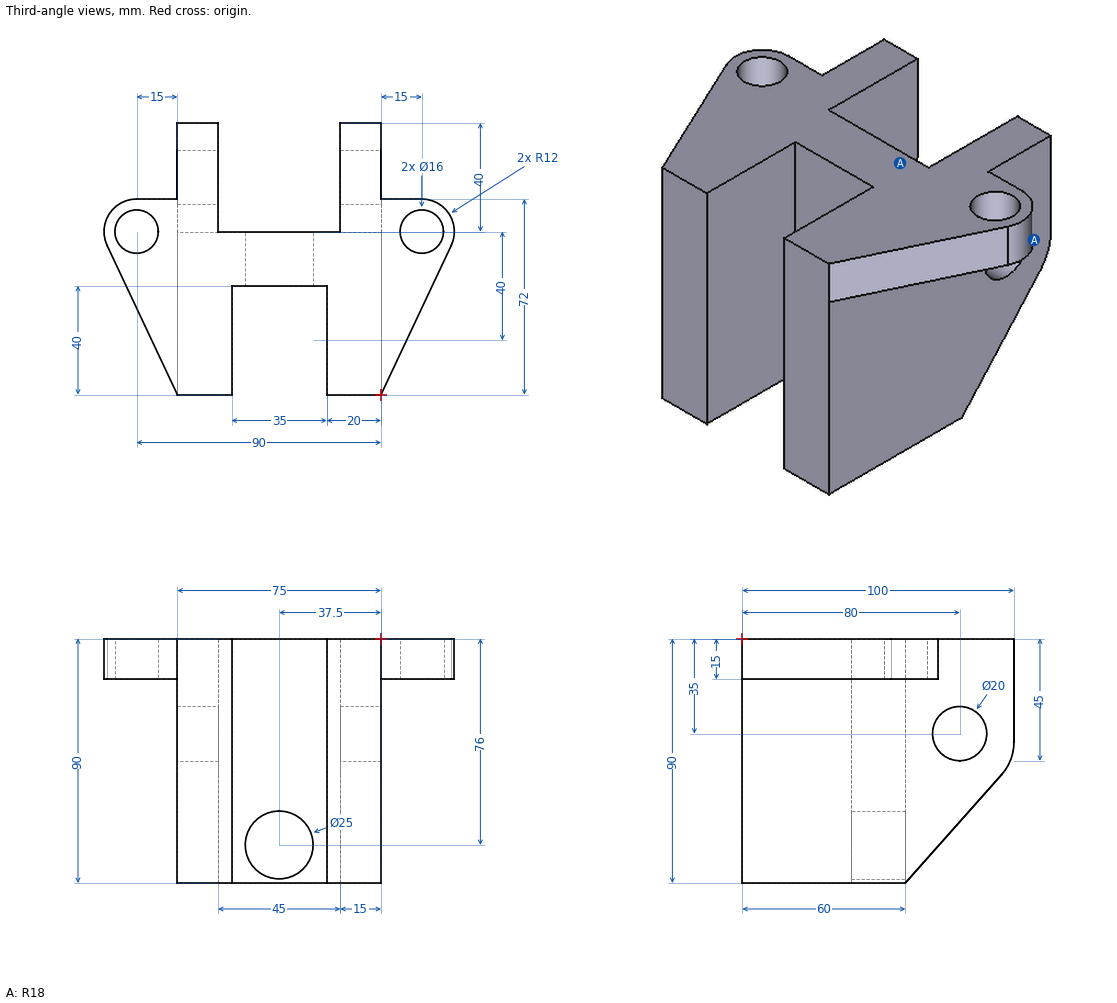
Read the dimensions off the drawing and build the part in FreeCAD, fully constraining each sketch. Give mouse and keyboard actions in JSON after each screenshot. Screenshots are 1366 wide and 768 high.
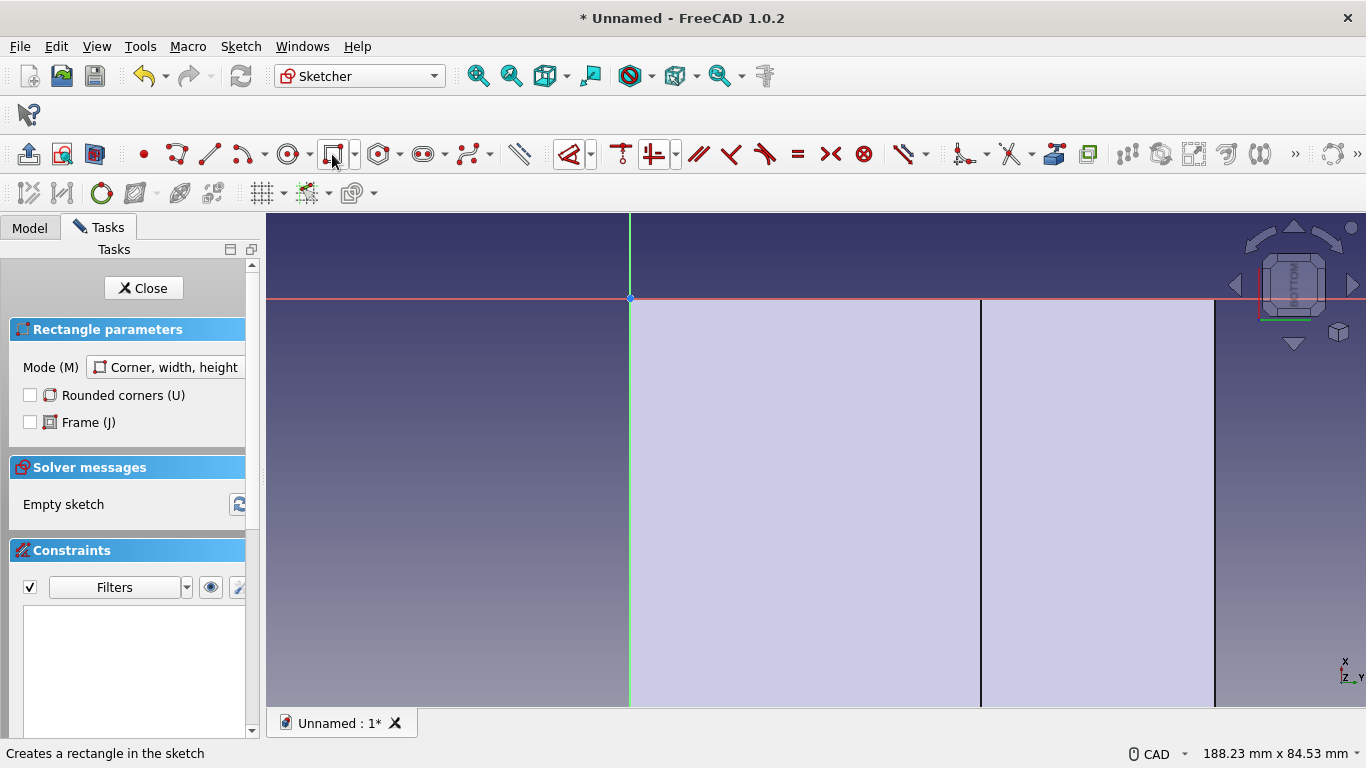
{"action": "left_click", "coordinate": [630, 416]}
{"action": "left_click", "coordinate": [864, 620]}
{"action": "key", "text": "Escape"}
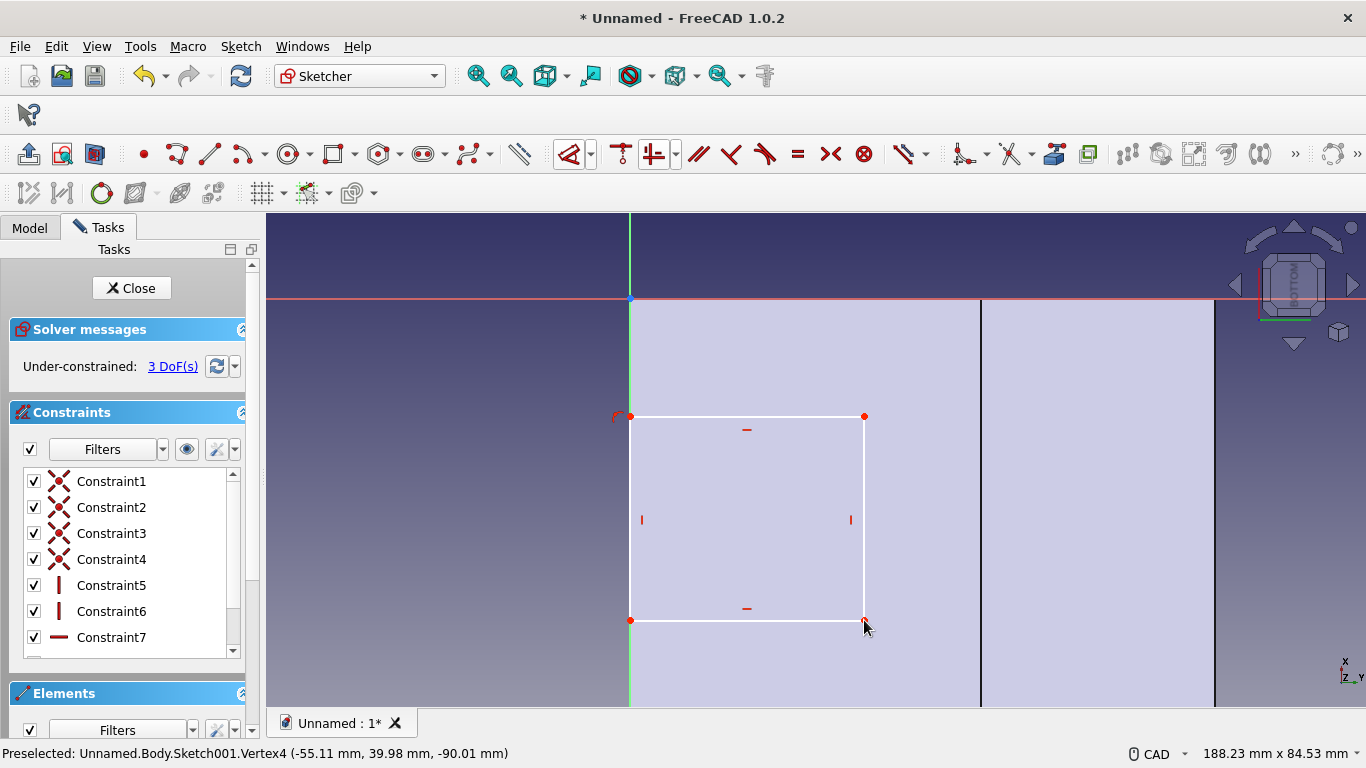
{"action": "left_click", "coordinate": [630, 478]}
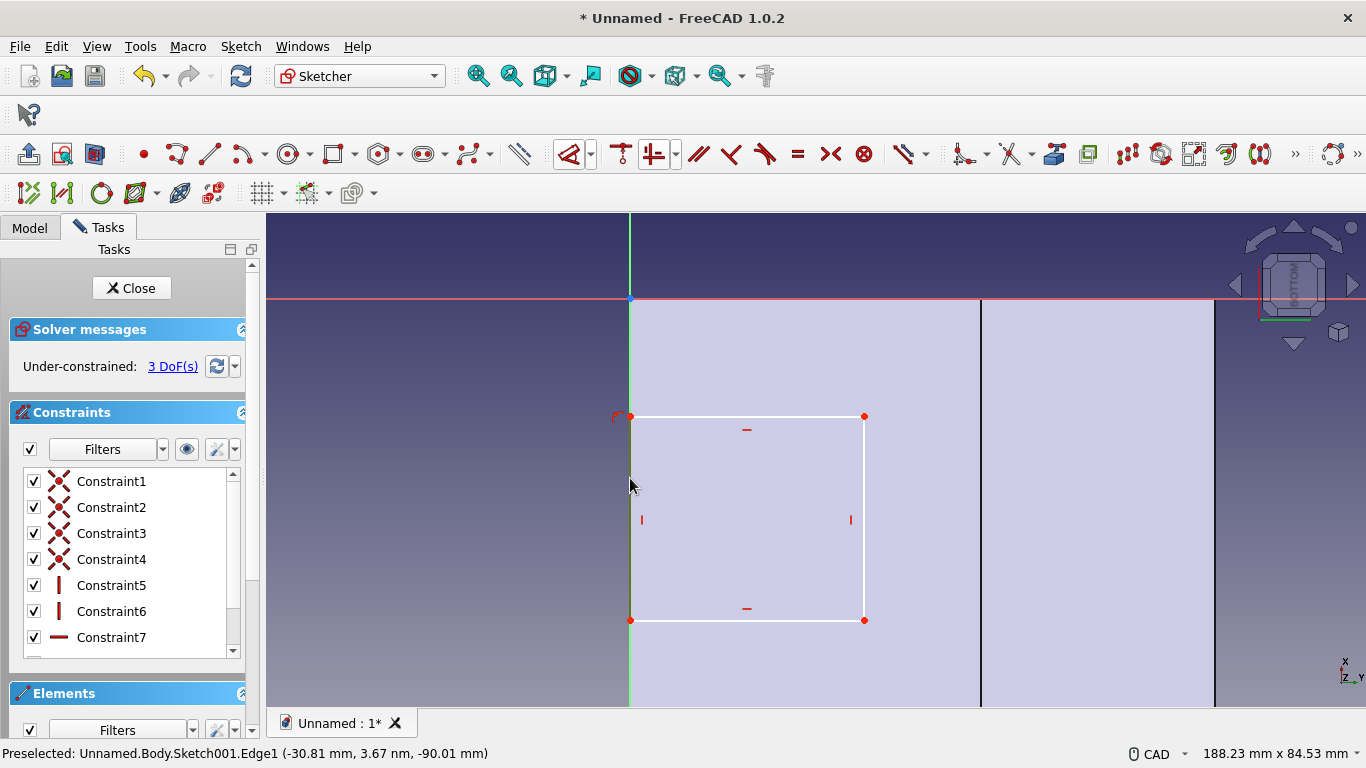
{"action": "key", "text": "i"}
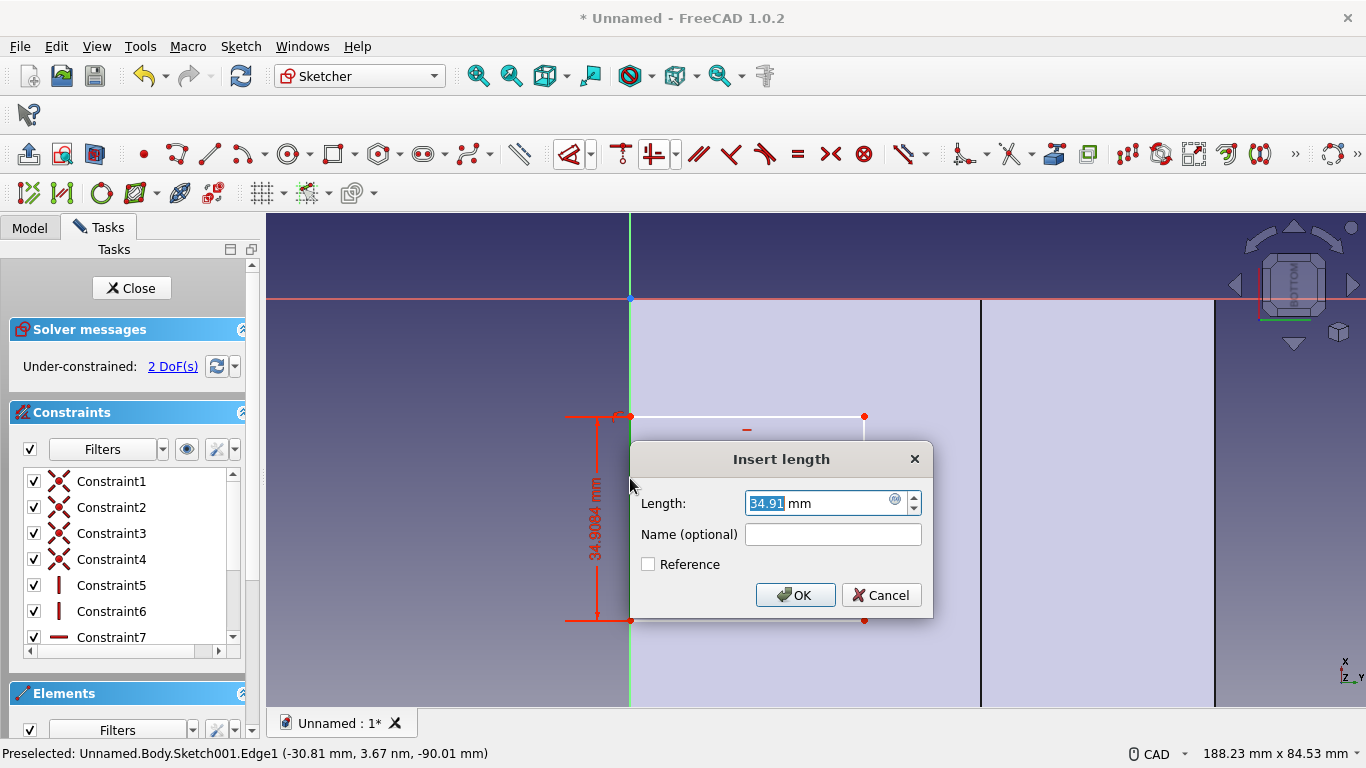
{"action": "type", "text": "35"}
{"action": "key", "text": "Return"}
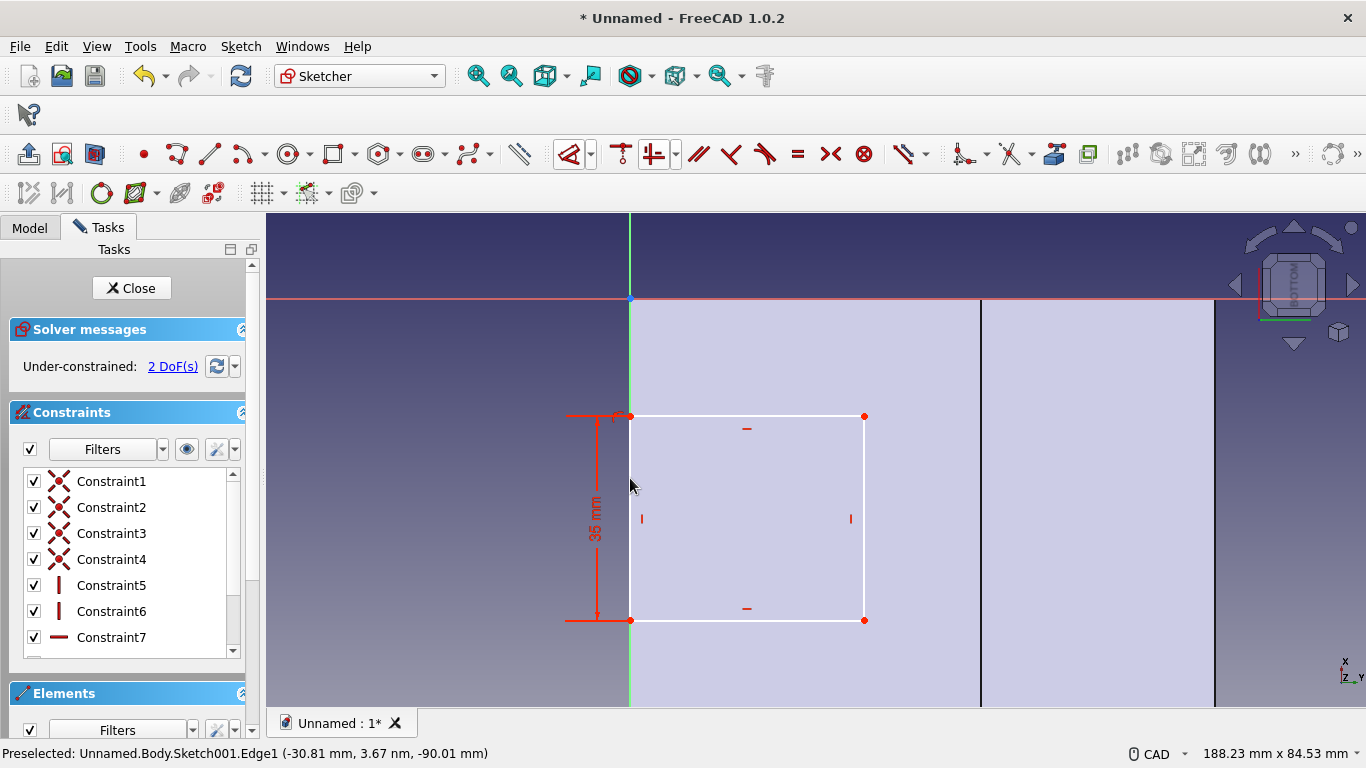
{"action": "left_click", "coordinate": [700, 621]}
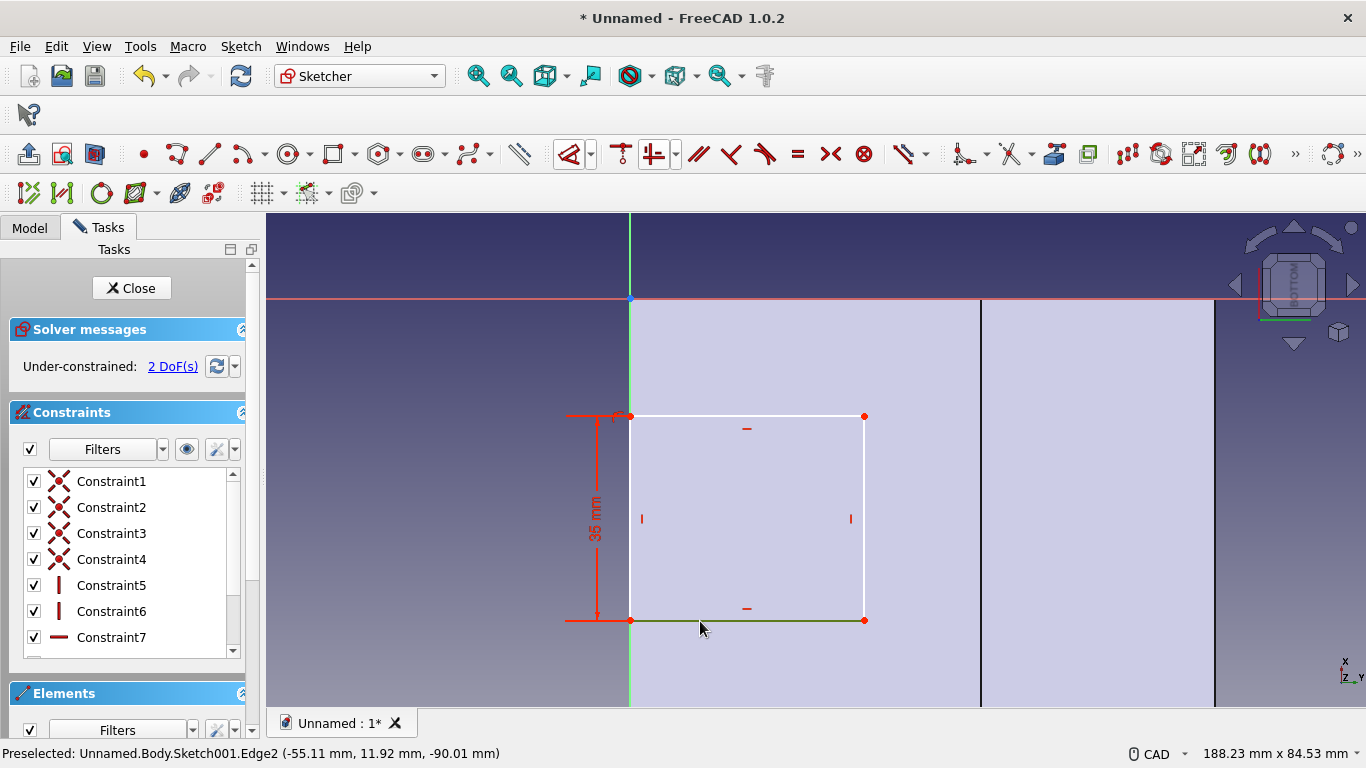
{"action": "key", "text": "l"}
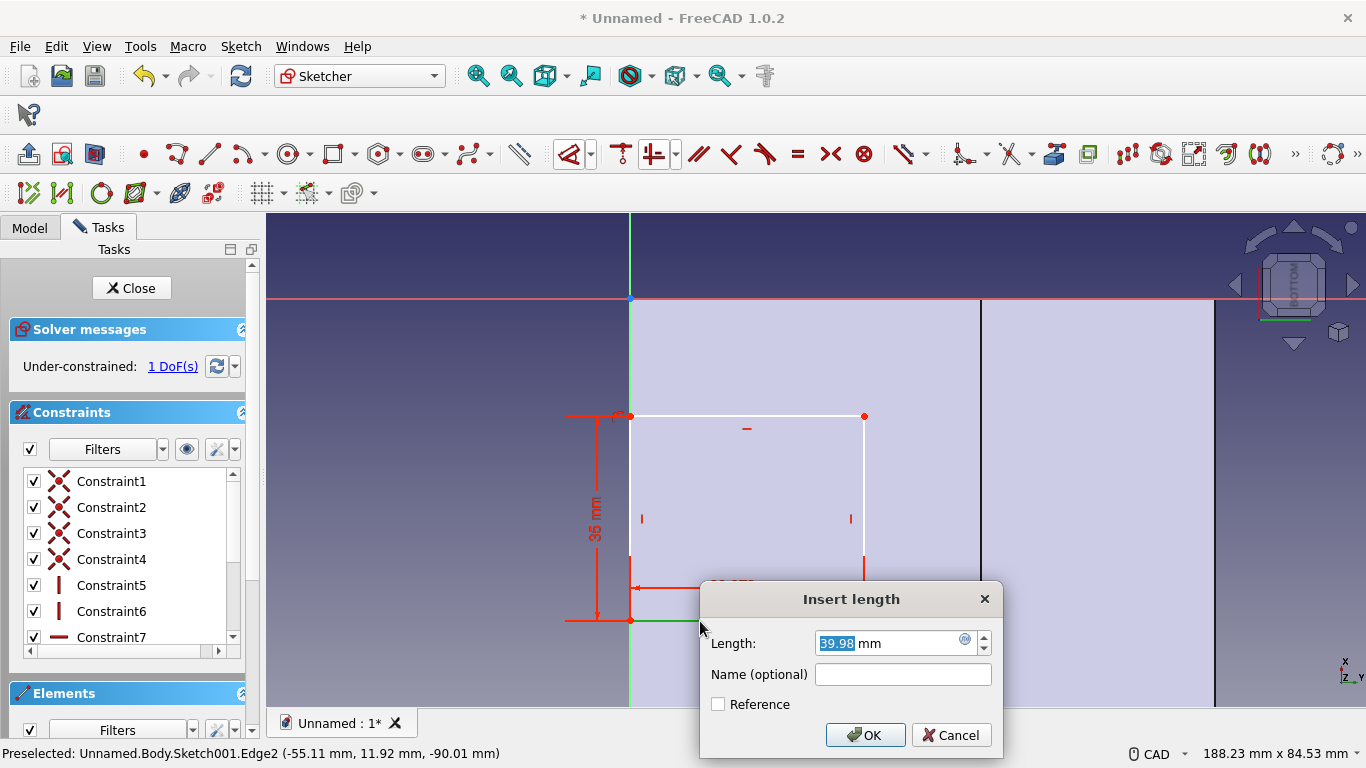
{"action": "type", "text": "40"}
{"action": "key", "text": "Return"}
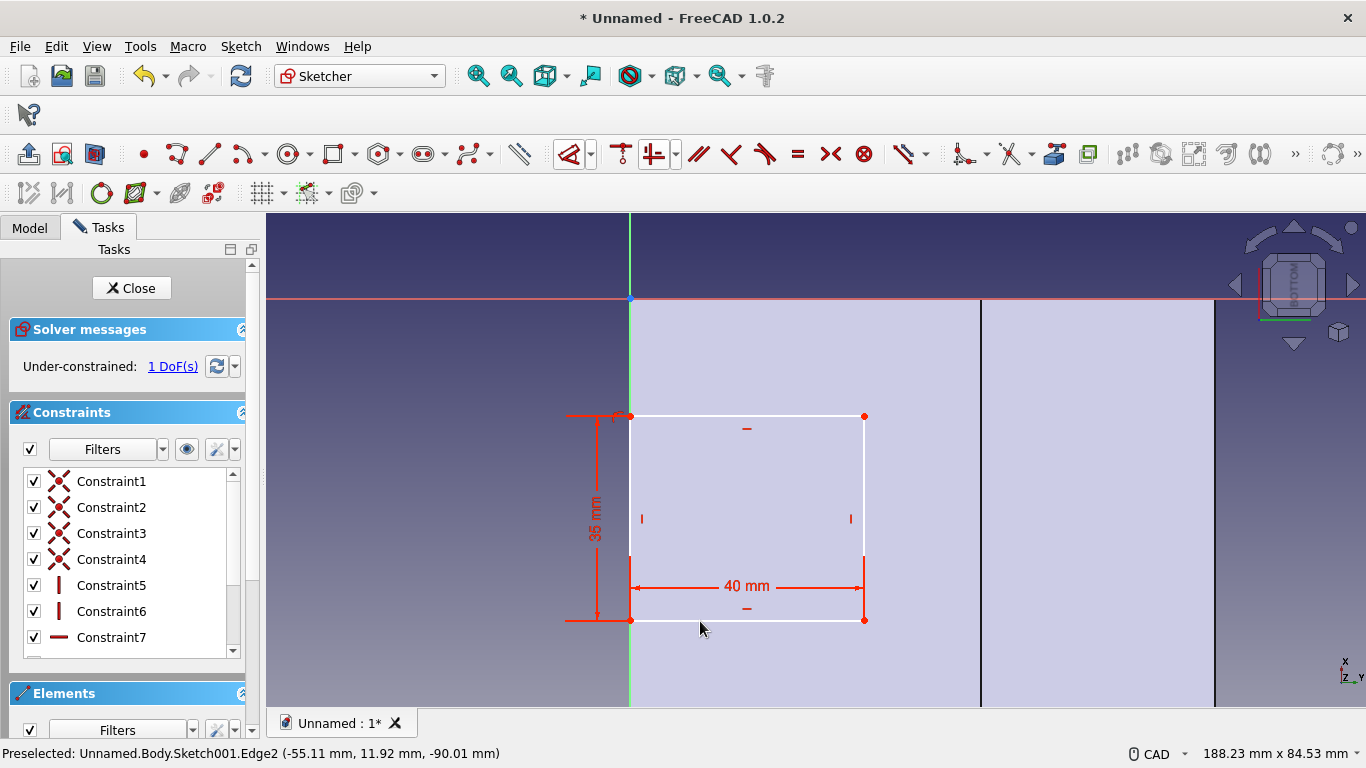
{"action": "left_click", "coordinate": [630, 416]}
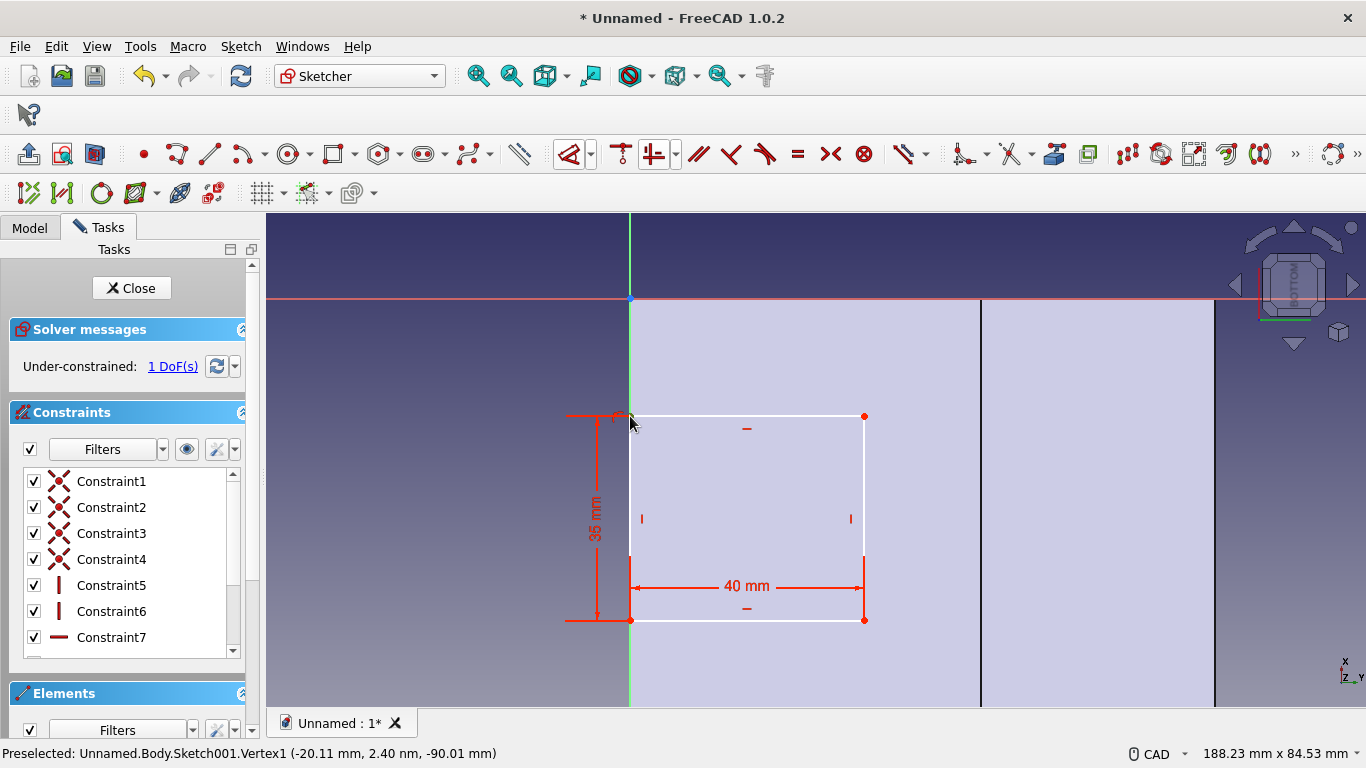
{"action": "left_click", "coordinate": [590, 154]}